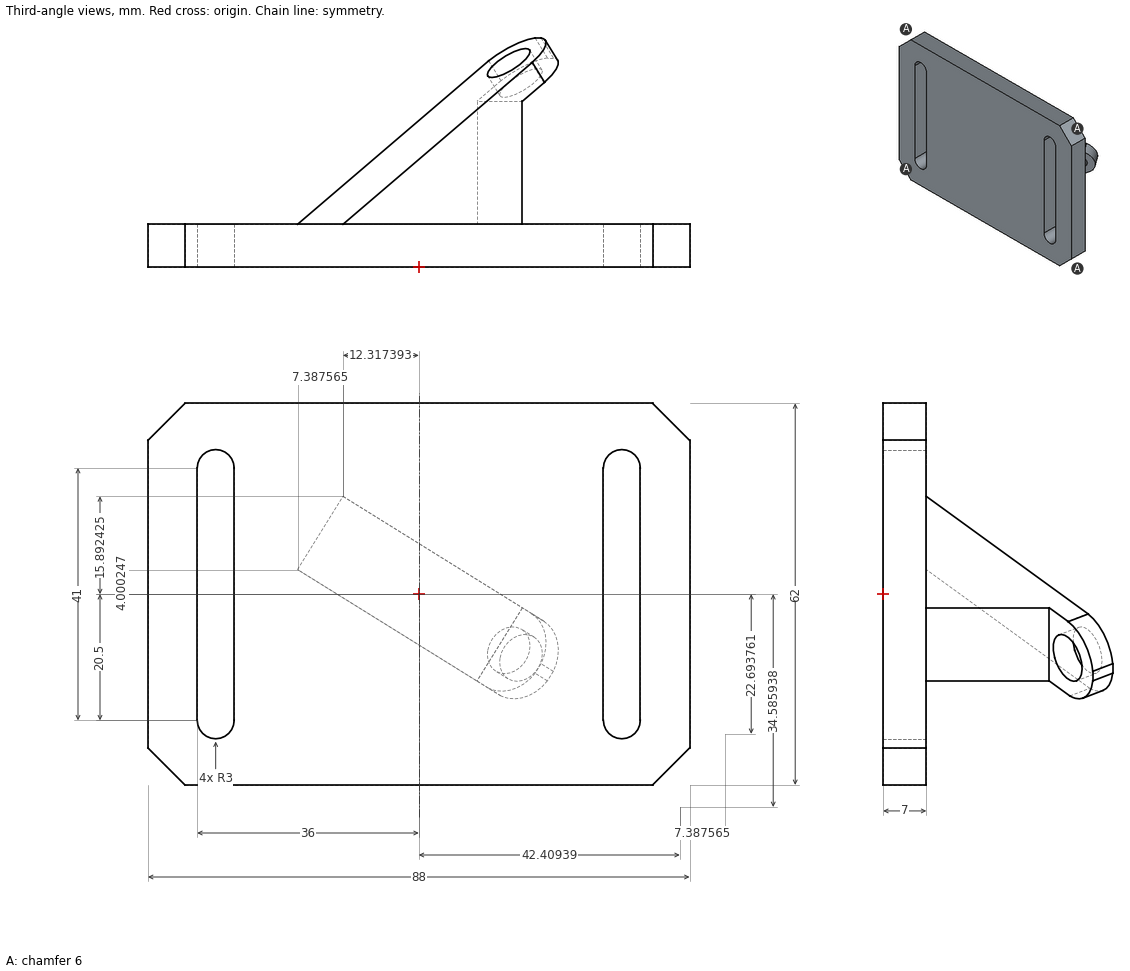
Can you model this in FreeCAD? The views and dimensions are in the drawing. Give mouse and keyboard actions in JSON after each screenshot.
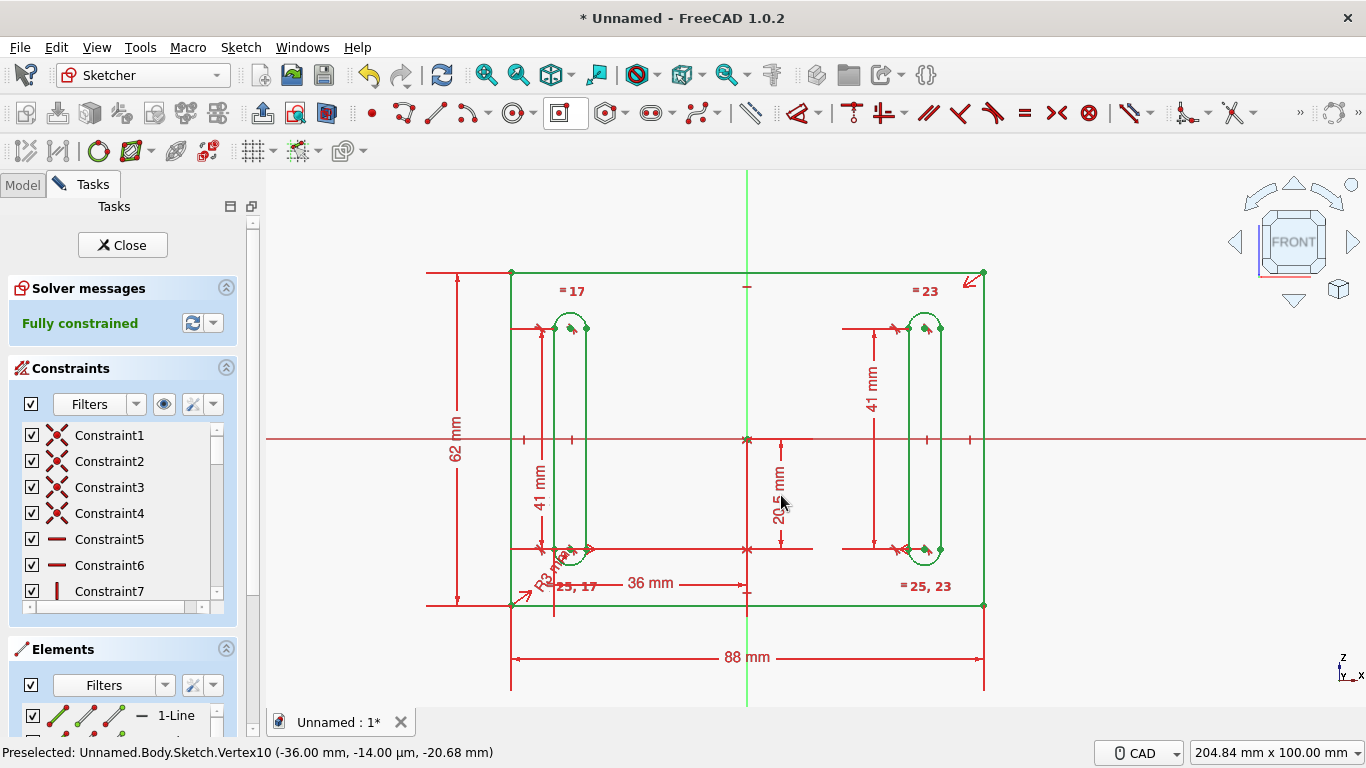
{"action": "left_click", "coordinate": [123, 245]}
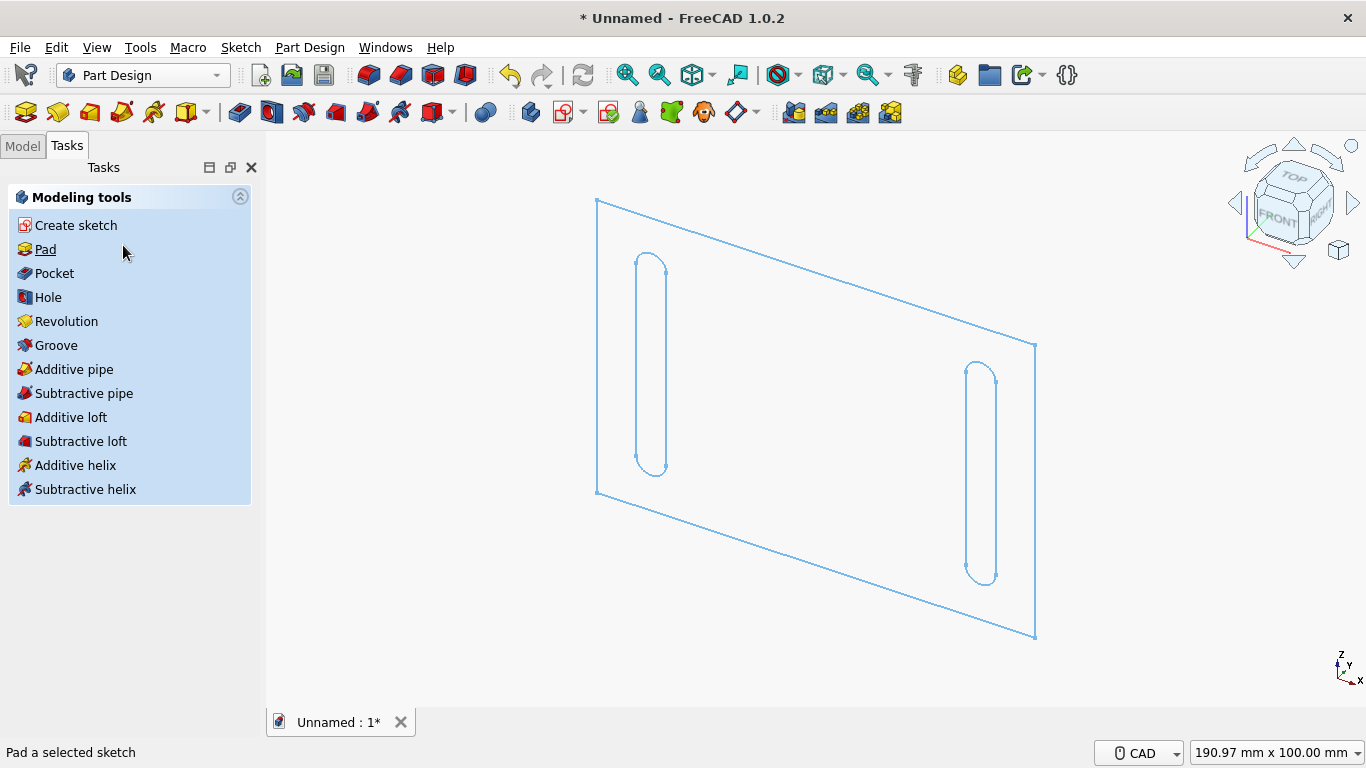
{"action": "left_click", "coordinate": [26, 112]}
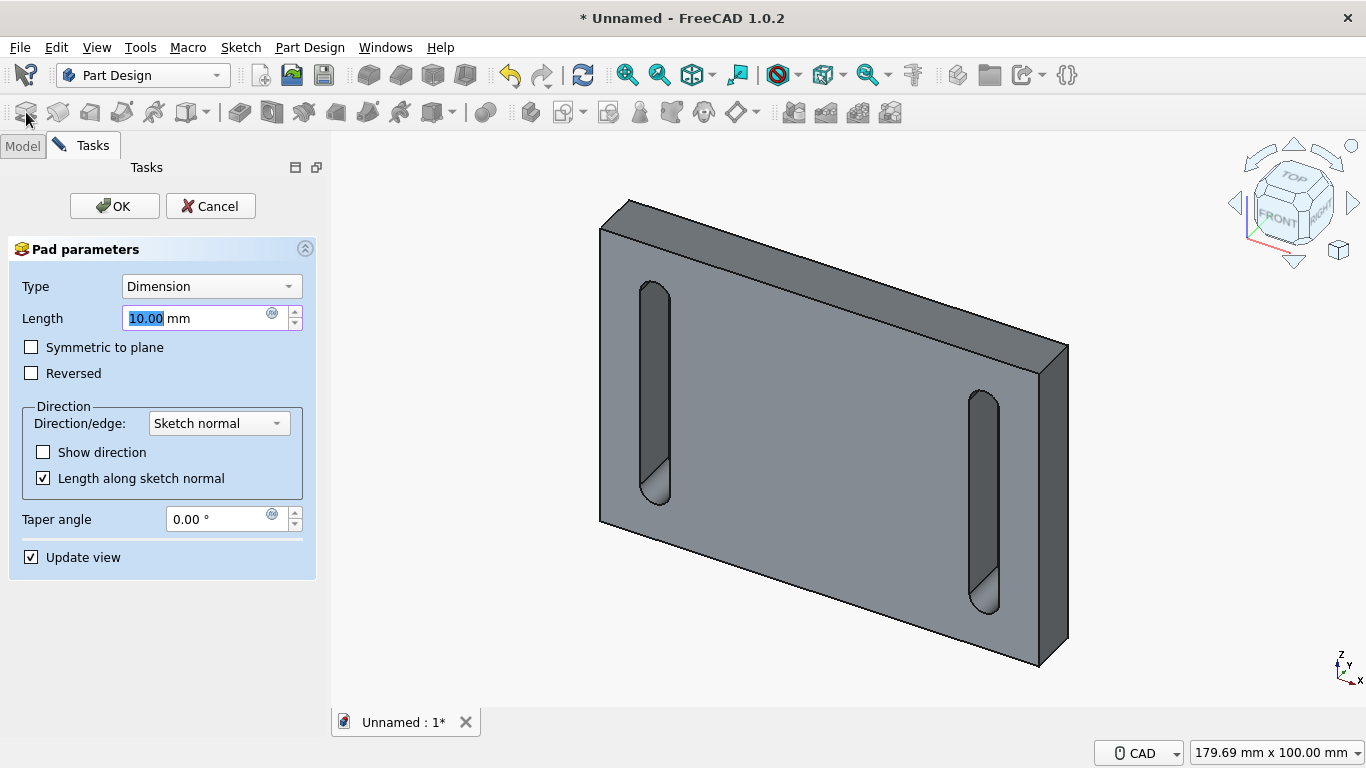
{"action": "type", "text": "7"}
{"action": "key", "text": "Tab"}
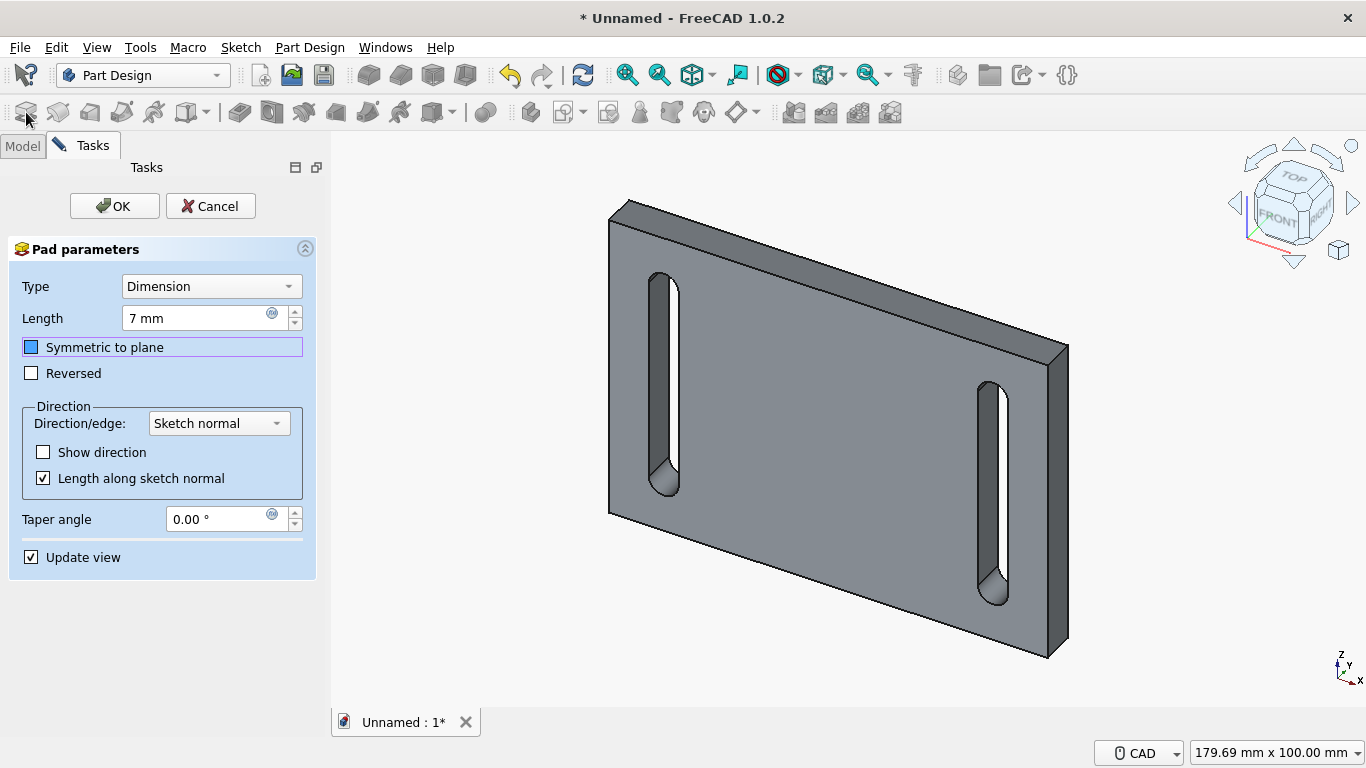
{"action": "left_click", "coordinate": [30, 373]}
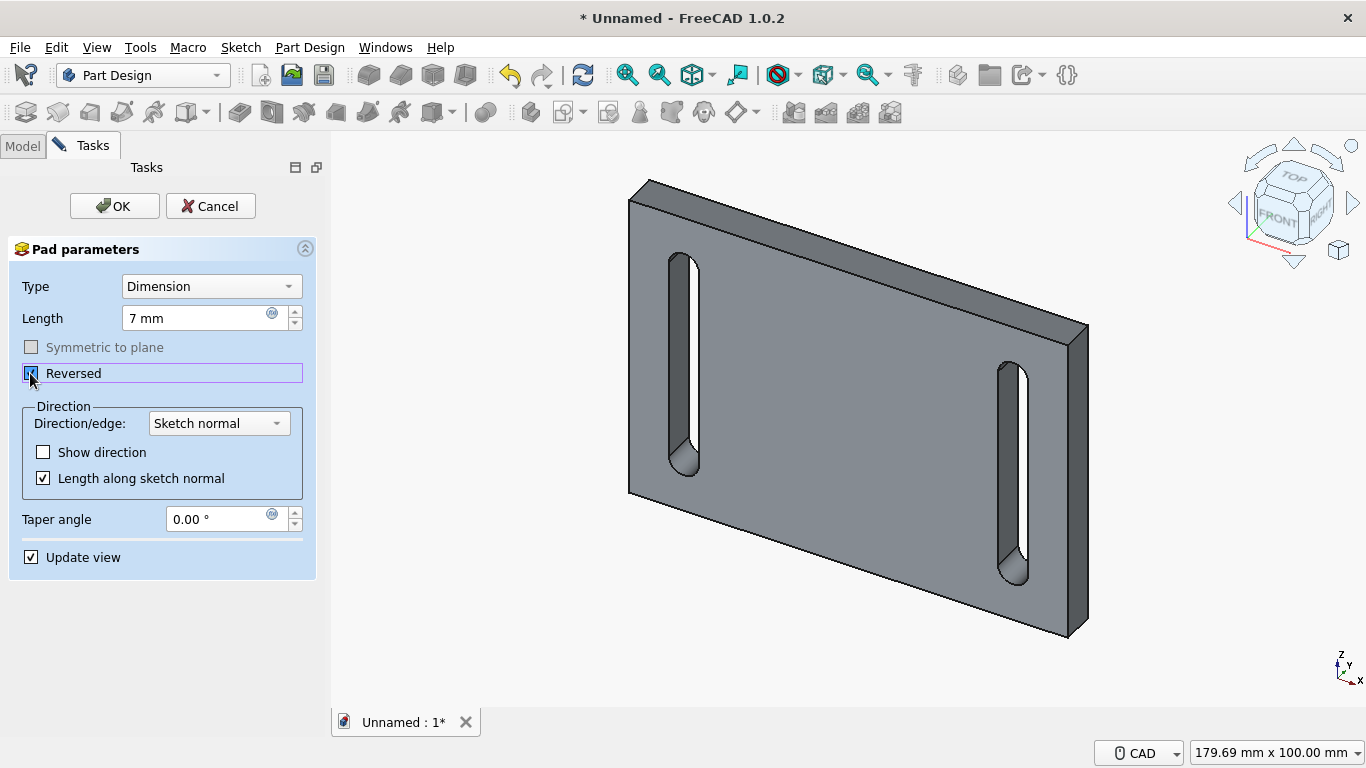
{"action": "left_click", "coordinate": [115, 206]}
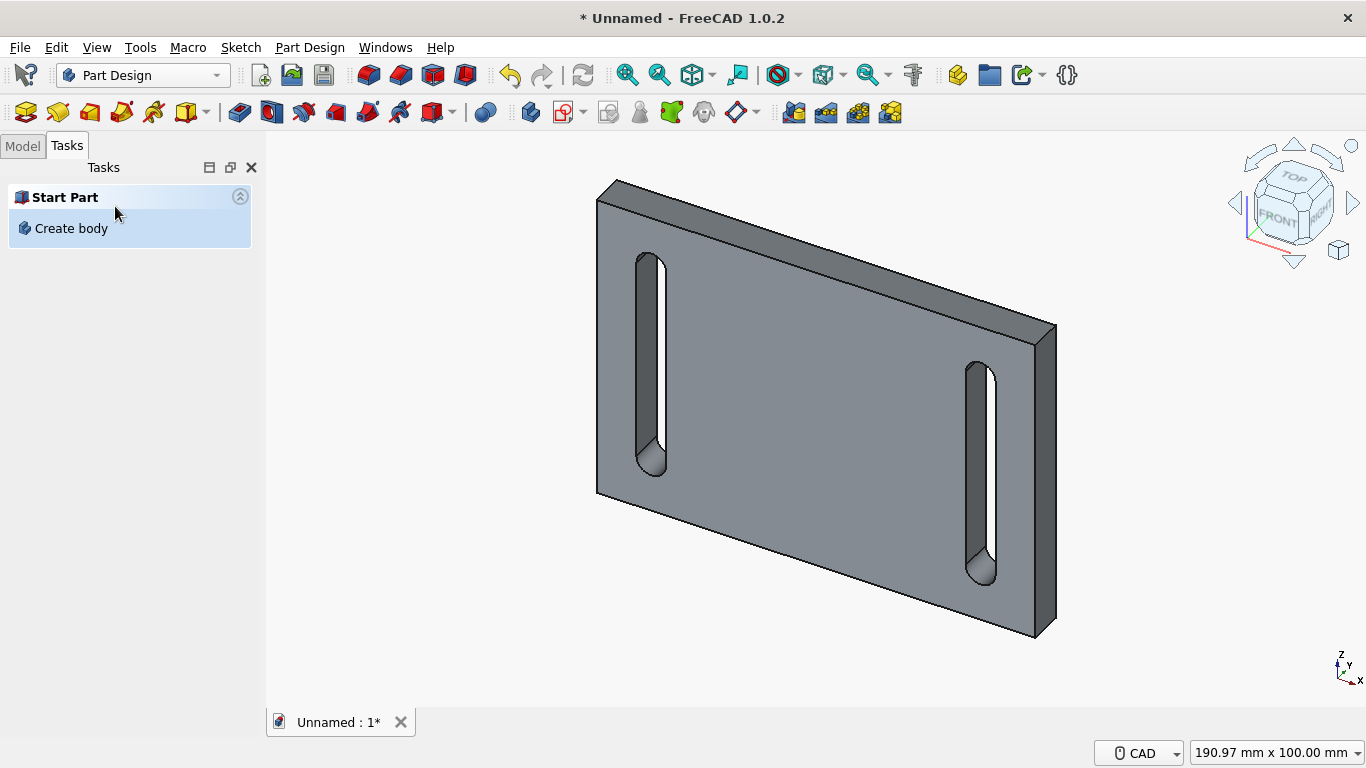
{"action": "left_click", "coordinate": [1046, 334]}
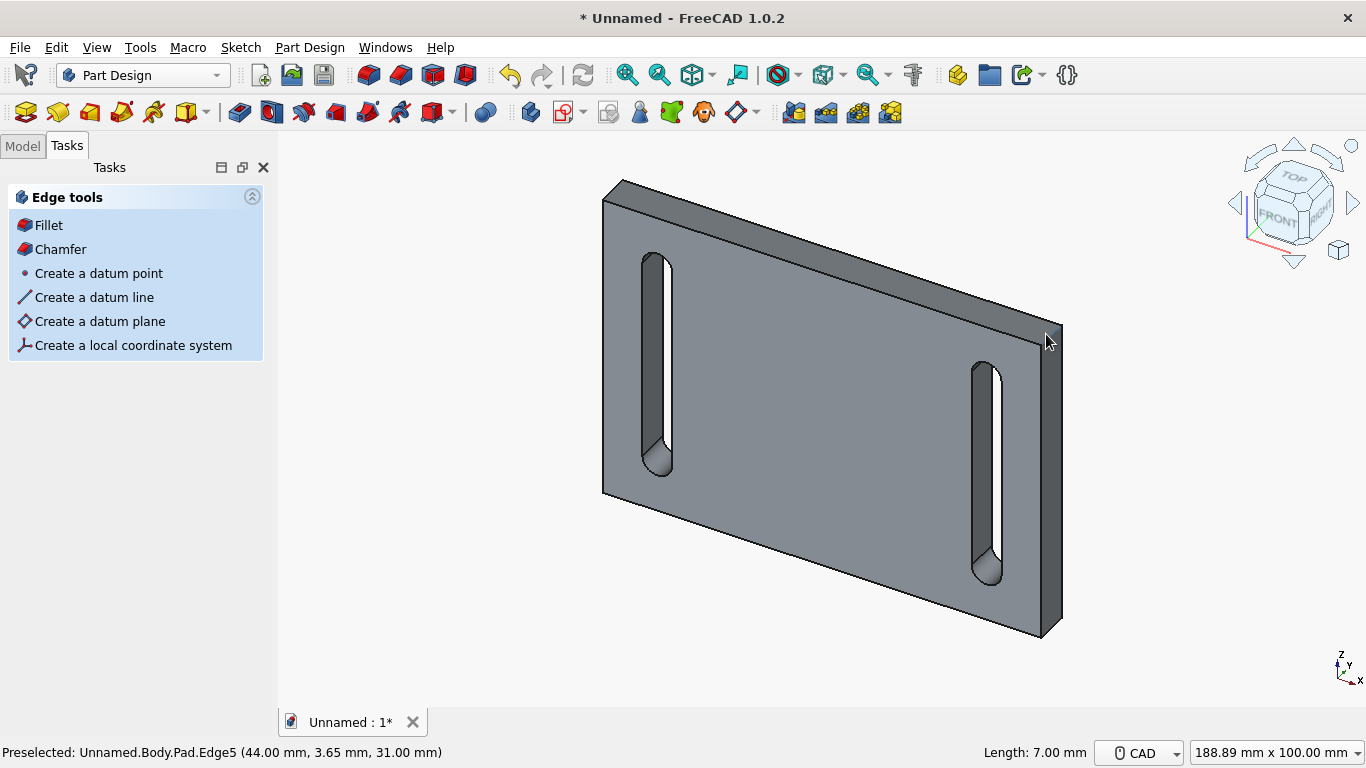
{"action": "key", "text": "0"}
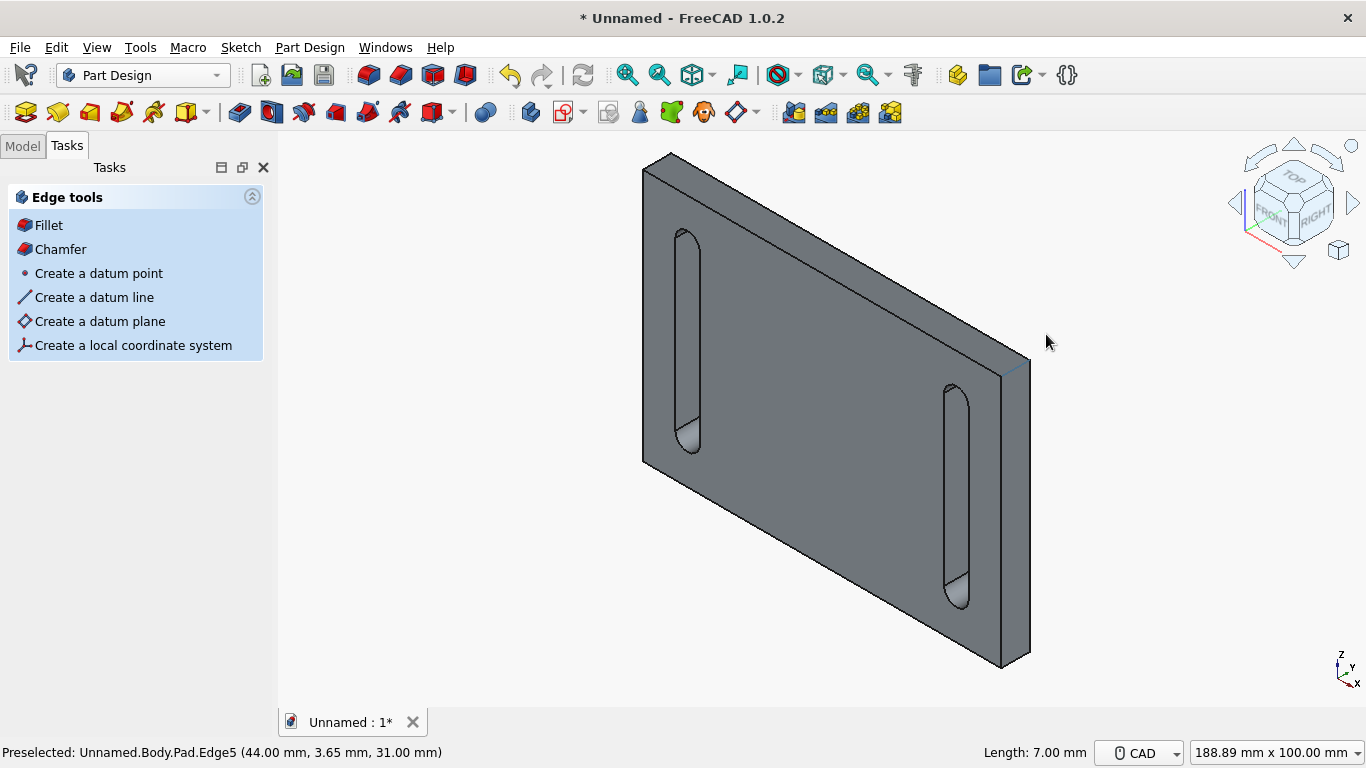
{"action": "key", "text": "2"}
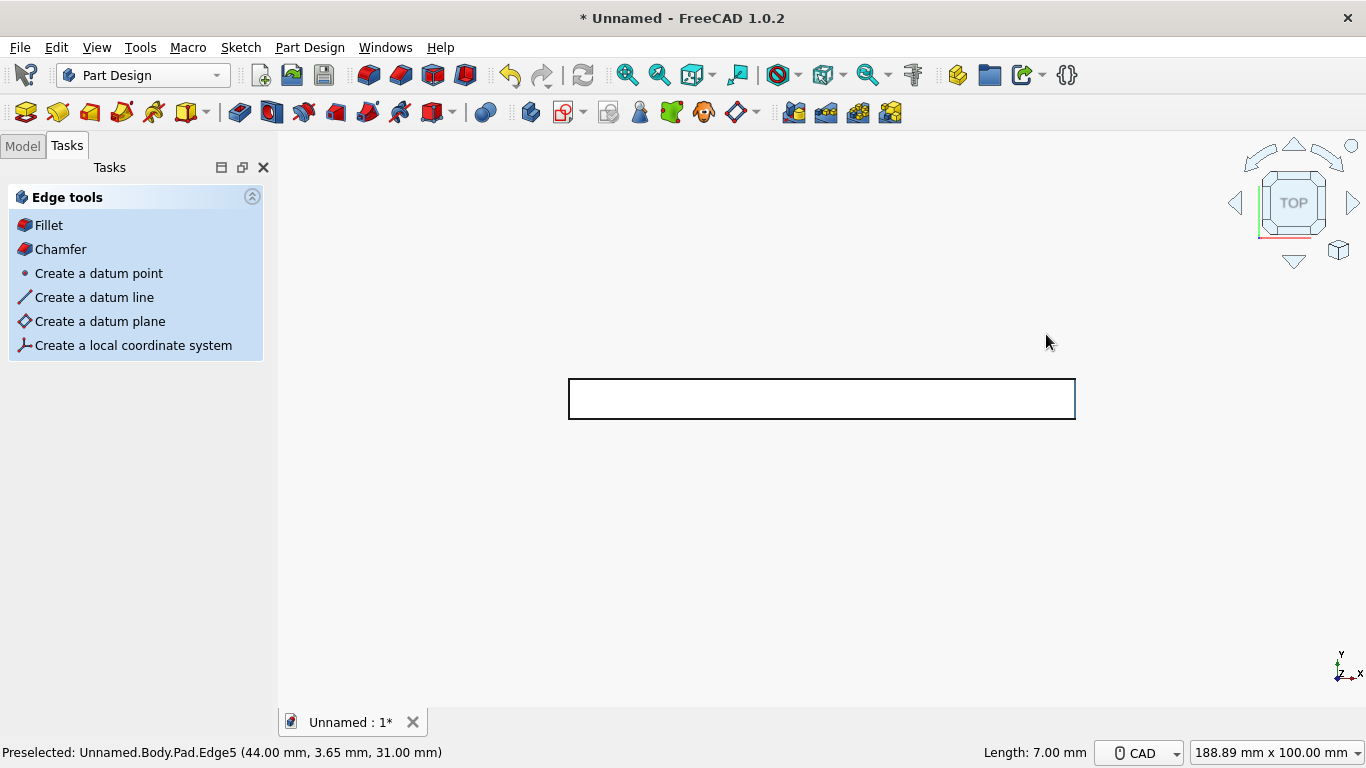
{"action": "left_click", "coordinate": [569, 398], "text": "ctrl"}